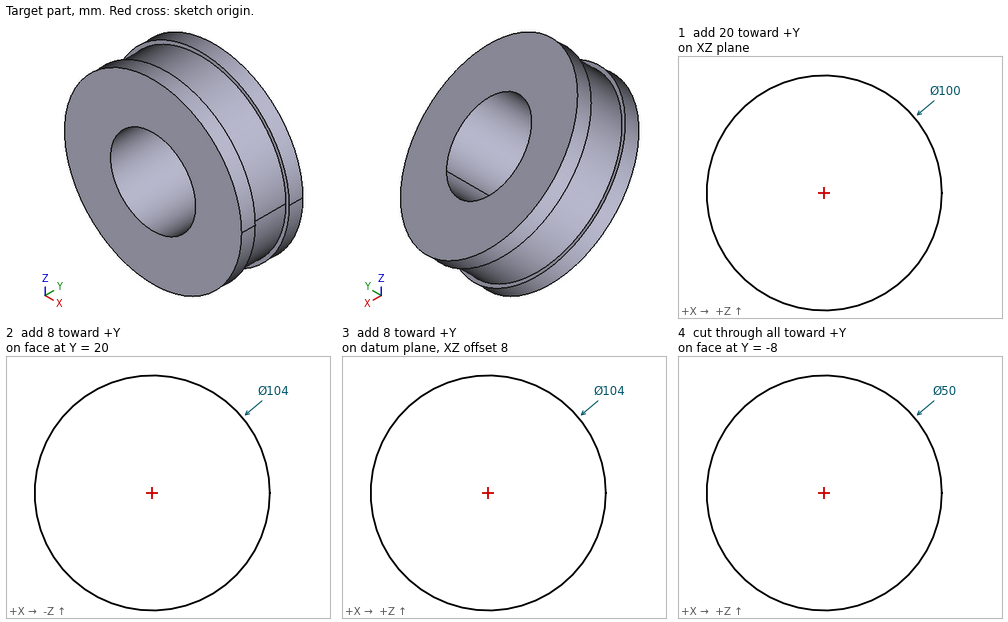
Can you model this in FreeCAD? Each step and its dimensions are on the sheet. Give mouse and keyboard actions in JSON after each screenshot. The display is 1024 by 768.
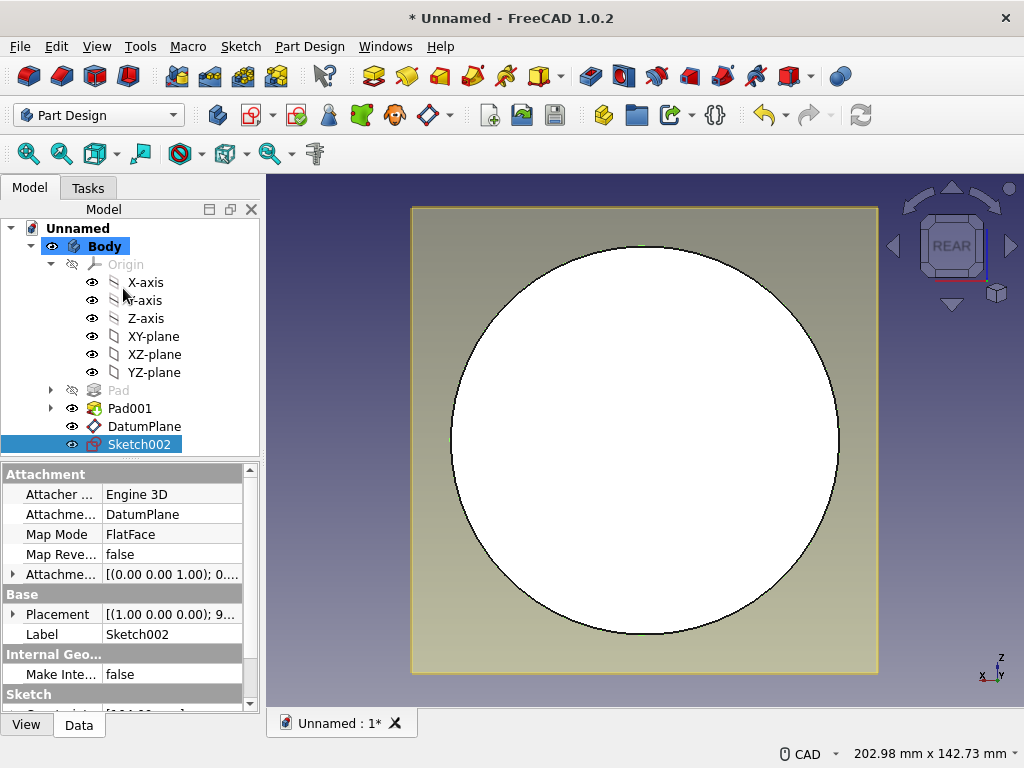
{"action": "left_click", "coordinate": [374, 76]}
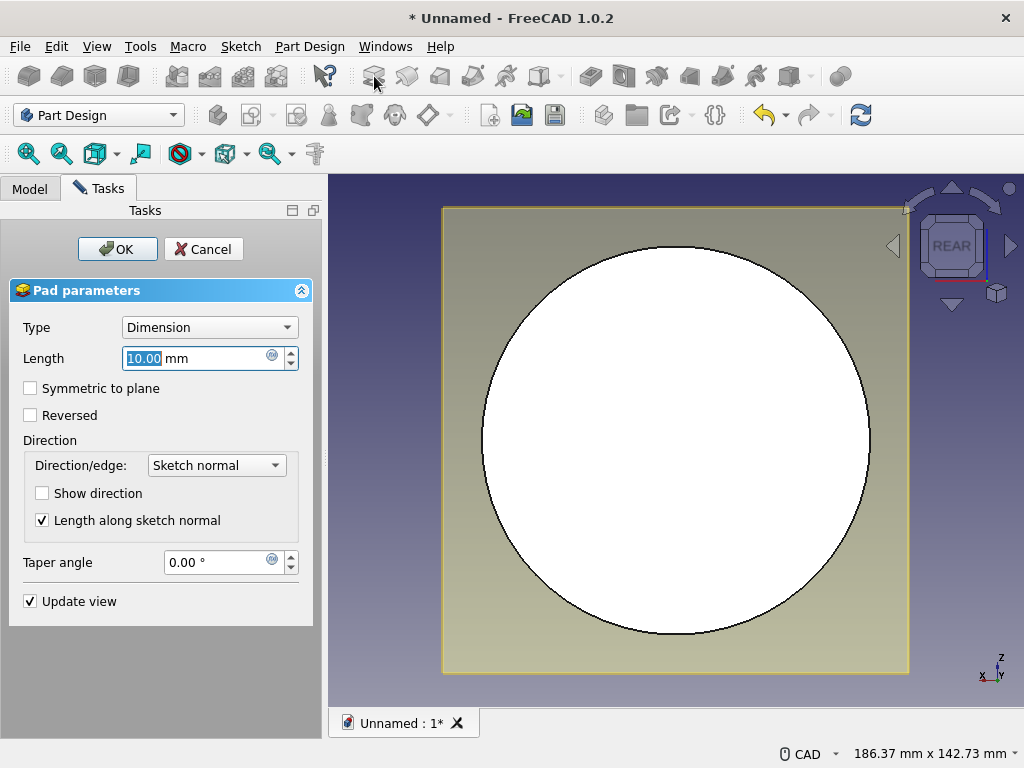
{"action": "type", "text": "8"}
{"action": "key", "text": "Tab"}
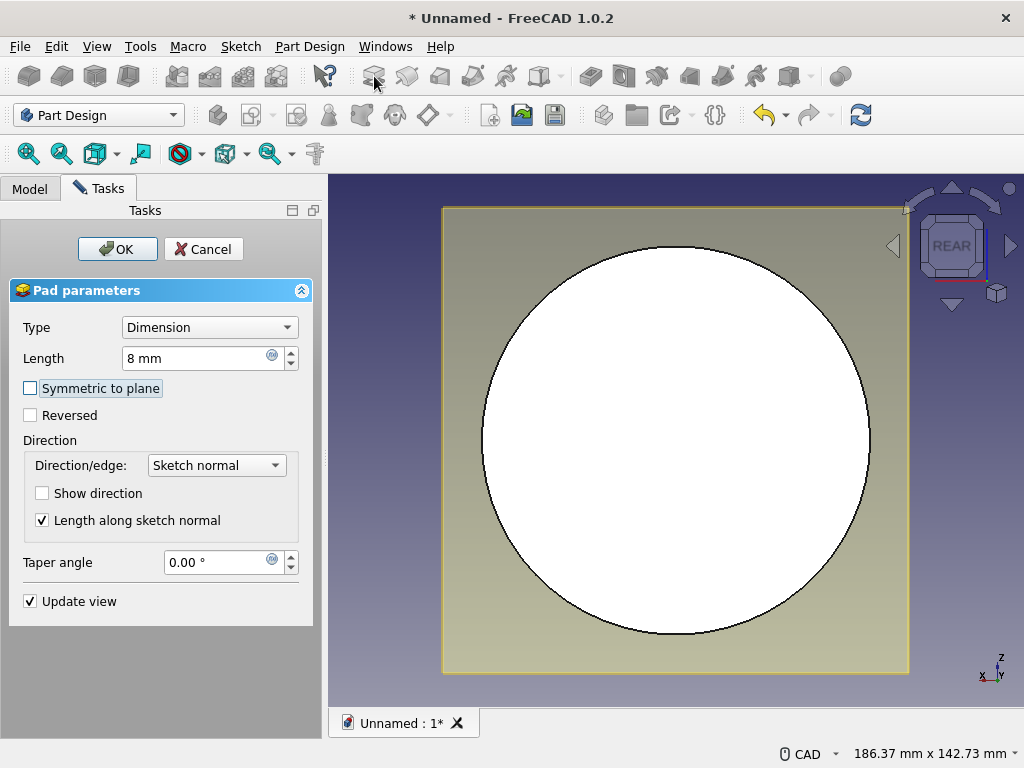
{"action": "left_click", "coordinate": [31, 415]}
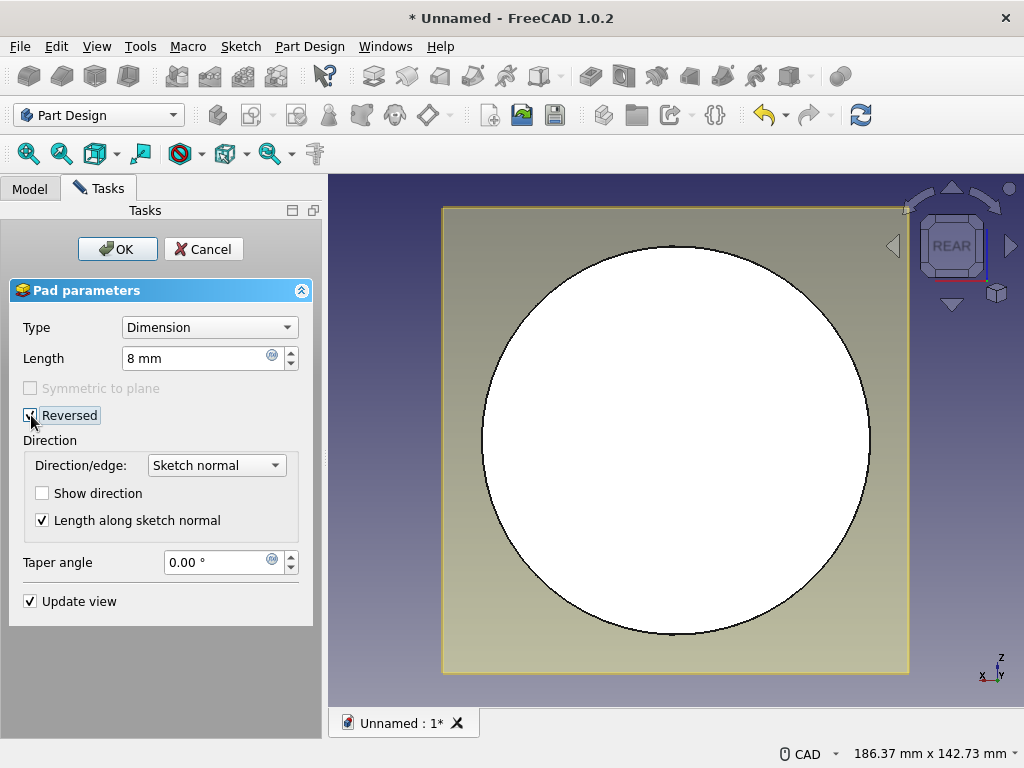
{"action": "left_click", "coordinate": [118, 249]}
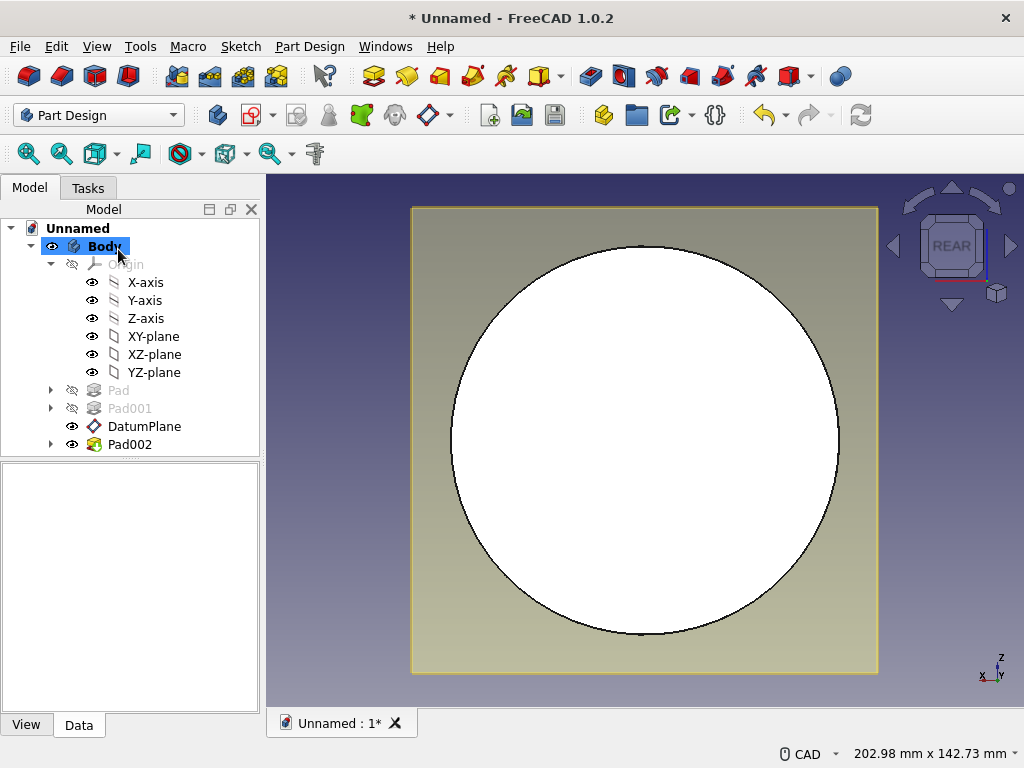
{"action": "left_click", "coordinate": [117, 426]}
{"action": "key", "text": "space"}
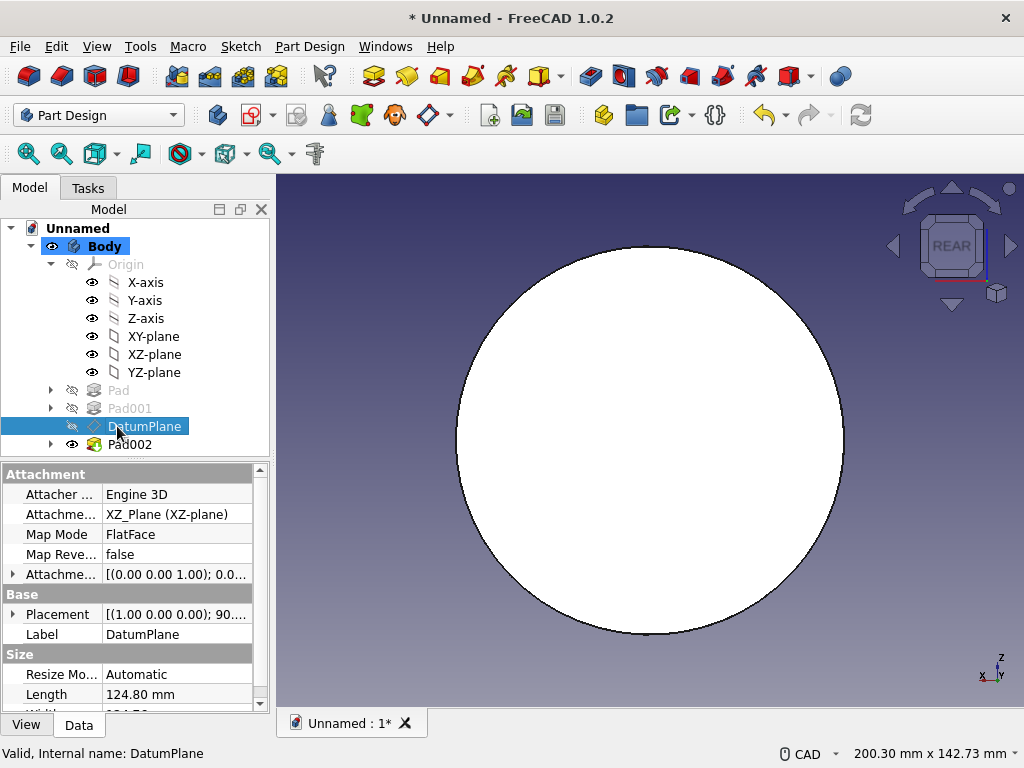
{"action": "key", "text": "0"}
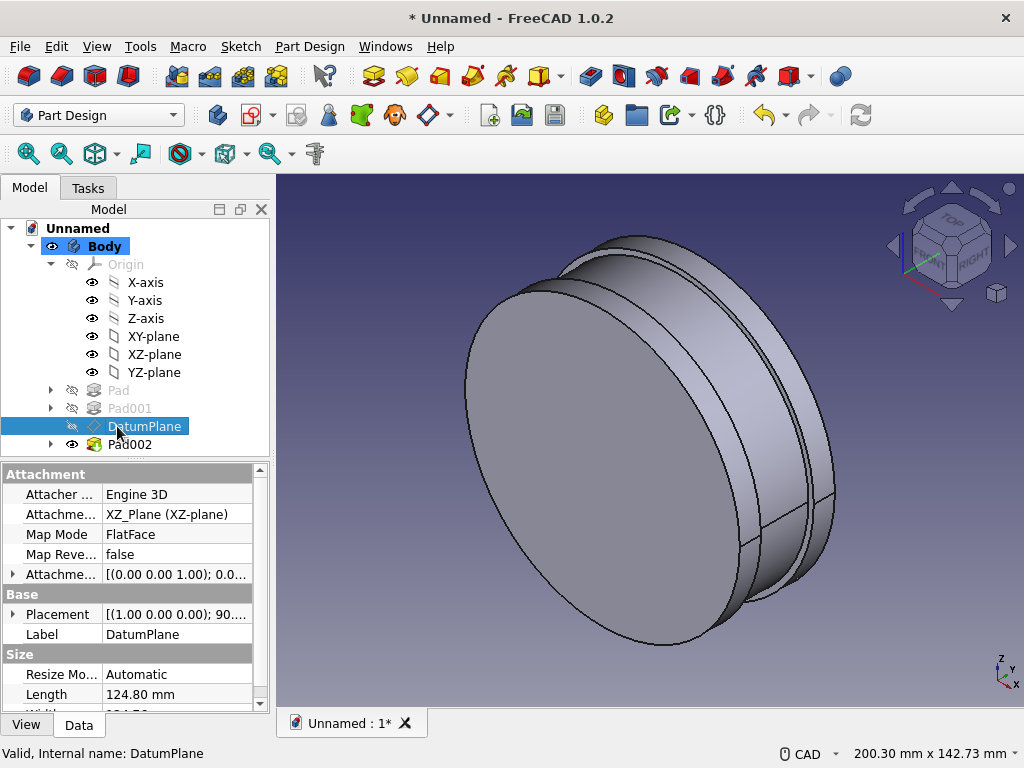
{"action": "left_click", "coordinate": [602, 467]}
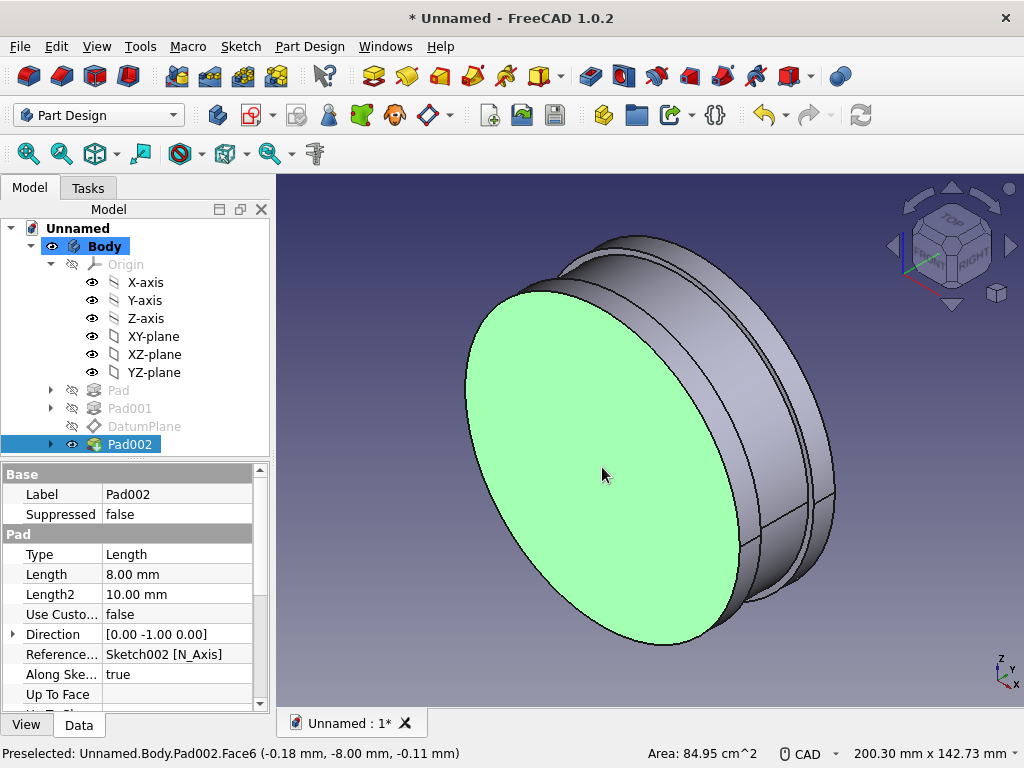
{"action": "left_click", "coordinate": [250, 116]}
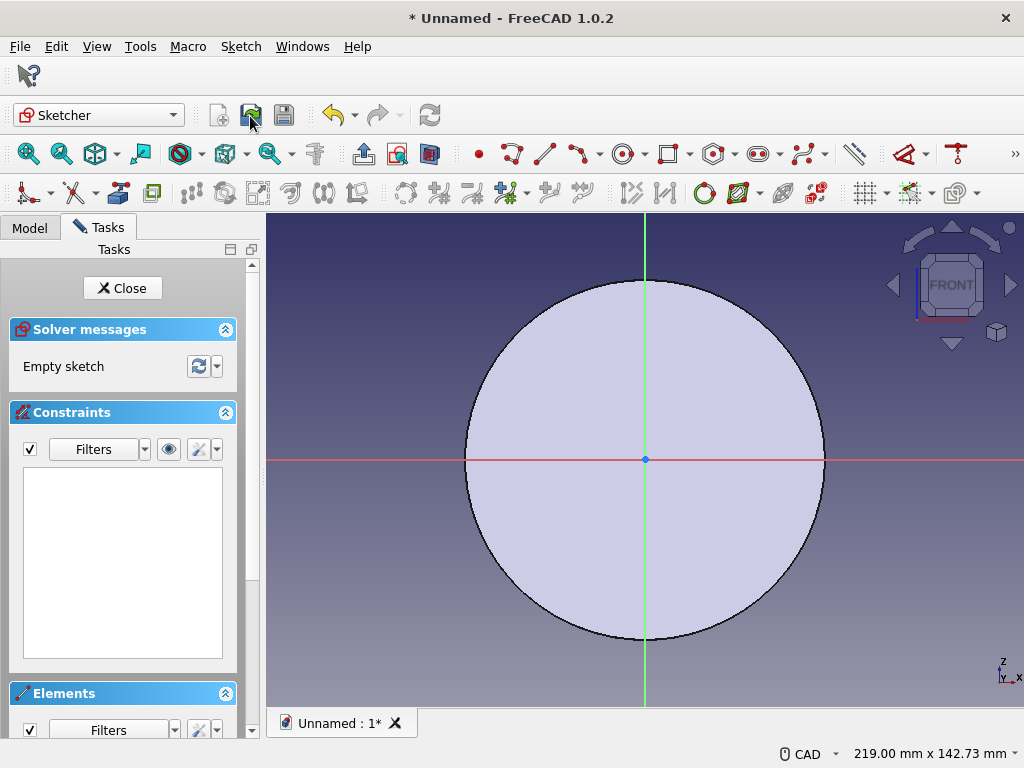
{"action": "scroll", "coordinate": [728, 460], "scroll_direction": "up", "scroll_amount": 3}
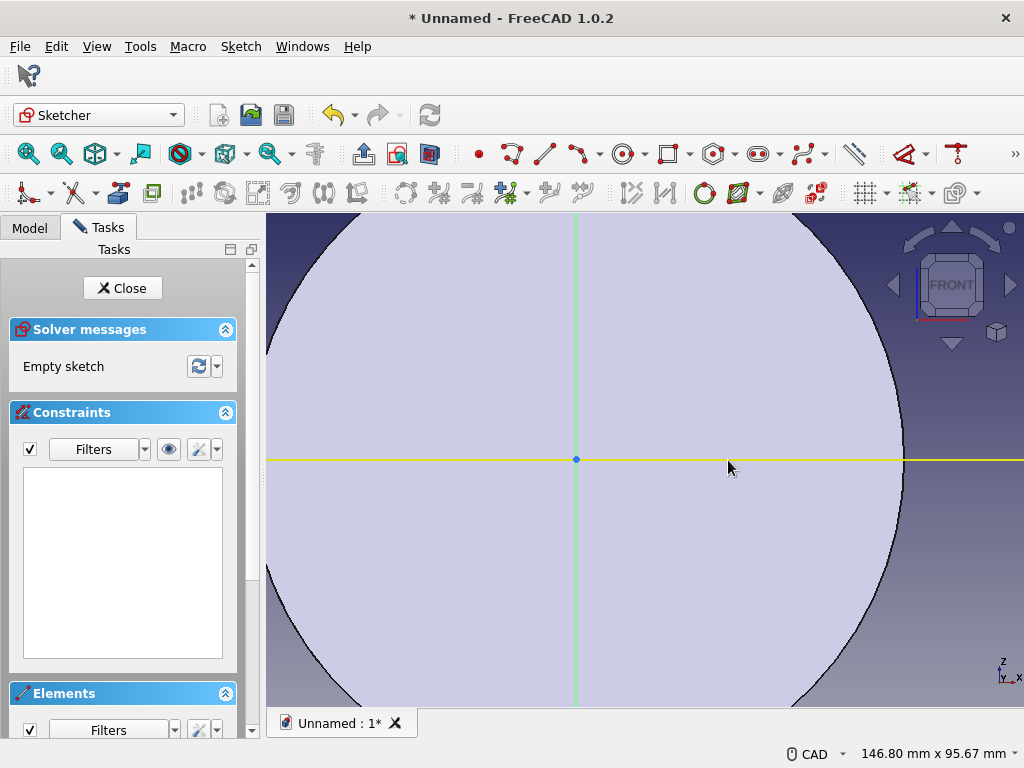
{"action": "key", "text": "g c"}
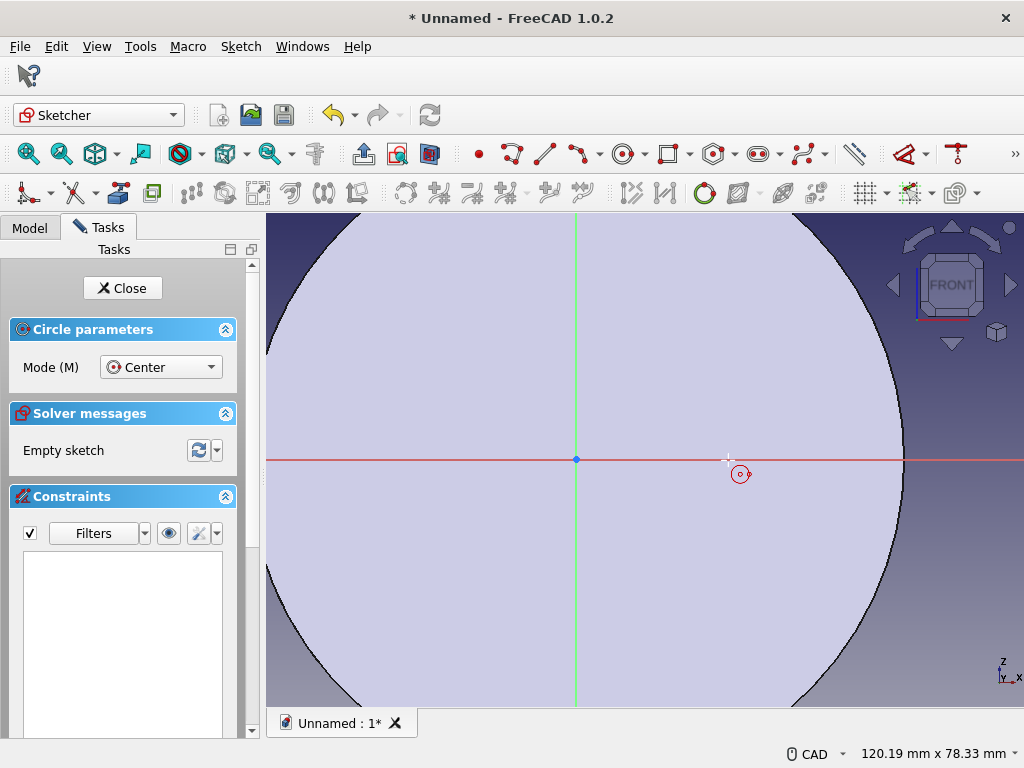
{"action": "left_click", "coordinate": [576, 460]}
{"action": "mouse_move", "coordinate": [688, 348]}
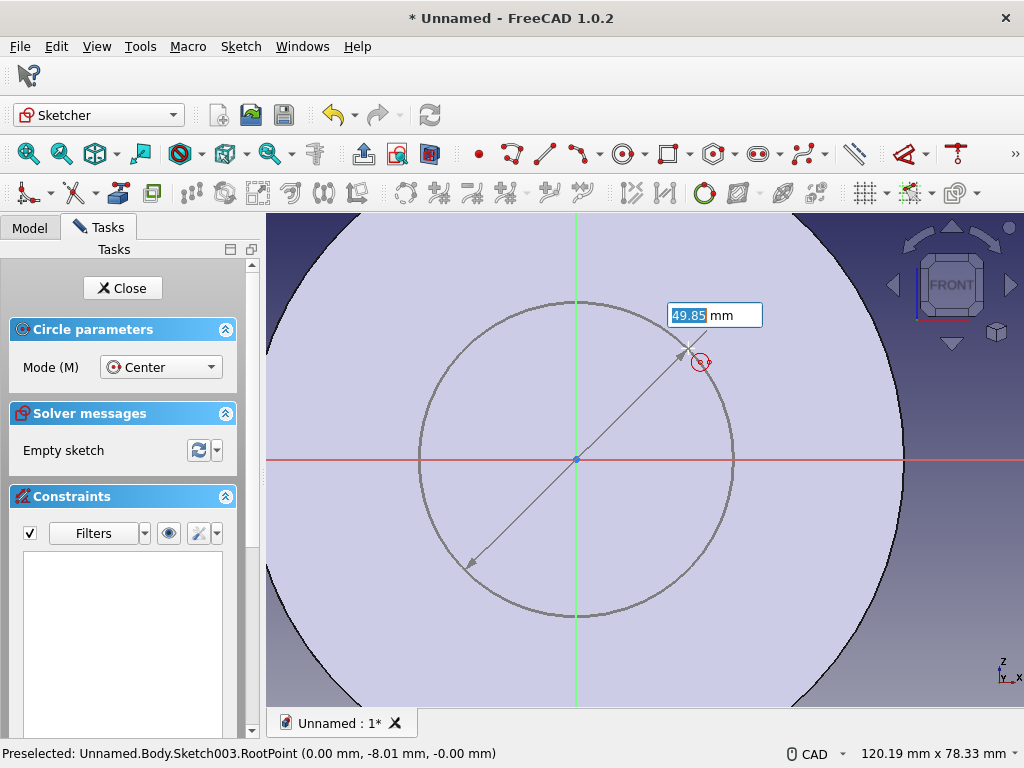
{"action": "type", "text": "50"}
{"action": "key", "text": "Return"}
{"action": "key", "text": "Escape"}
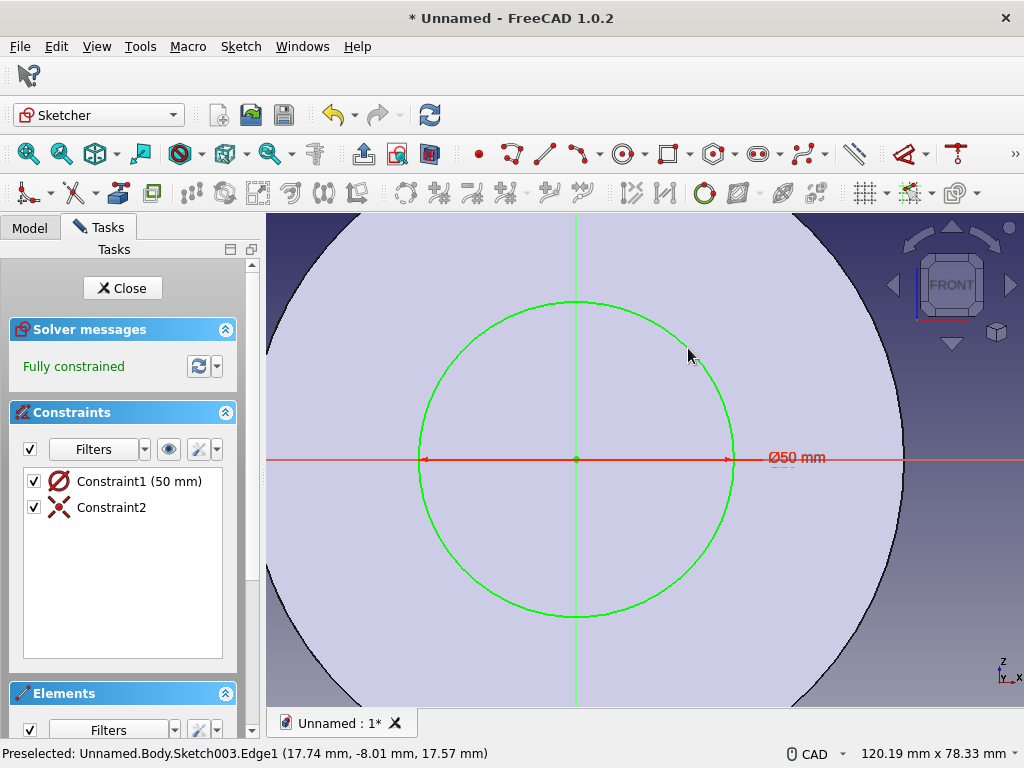
{"action": "left_click", "coordinate": [123, 288]}